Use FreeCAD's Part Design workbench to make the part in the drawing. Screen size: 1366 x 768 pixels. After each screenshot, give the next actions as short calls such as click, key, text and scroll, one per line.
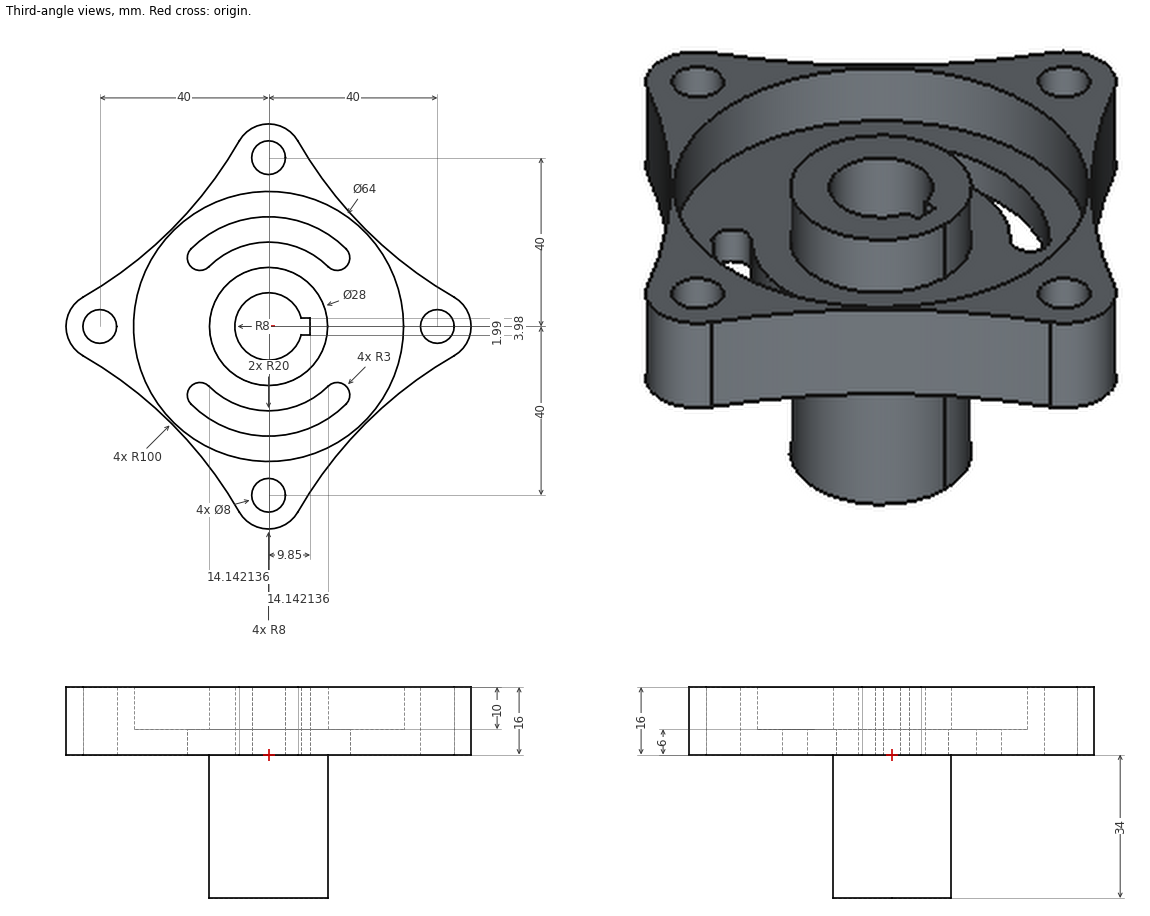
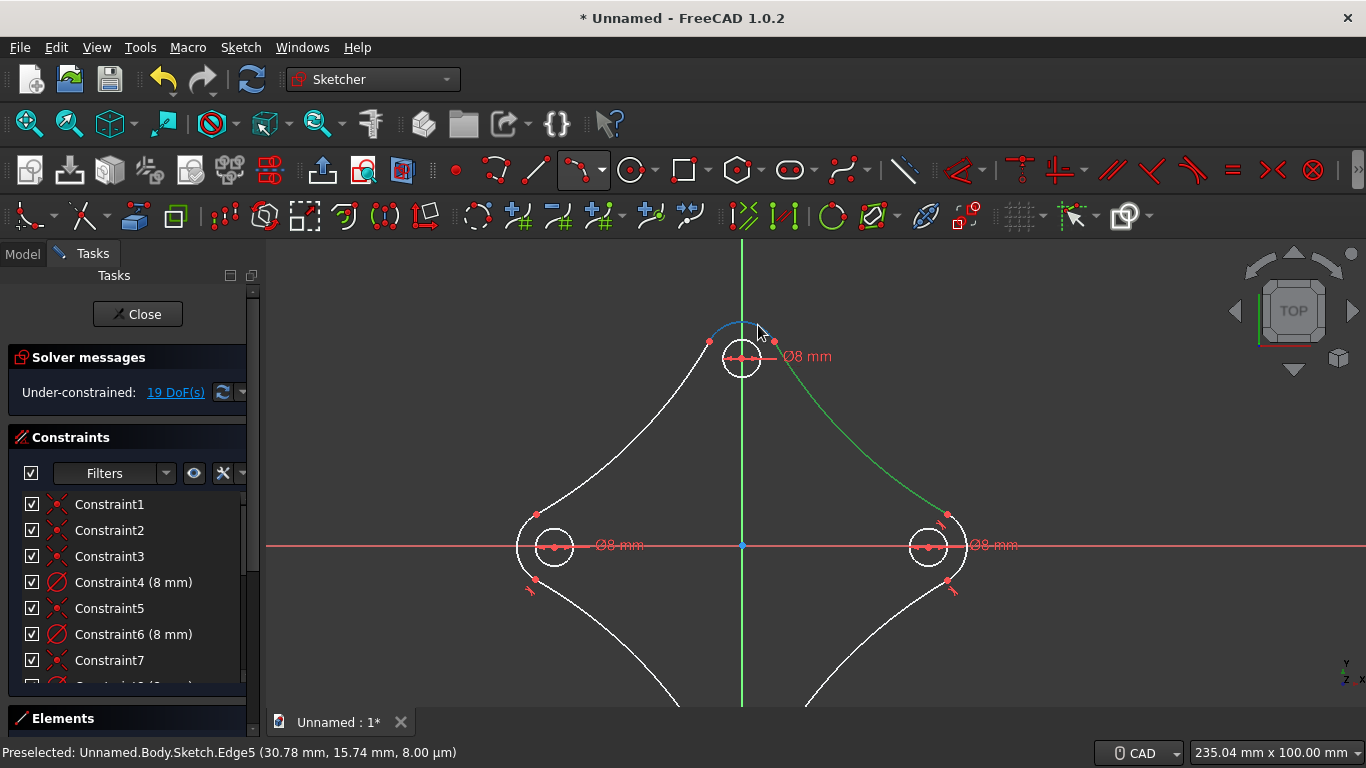
click(757, 325)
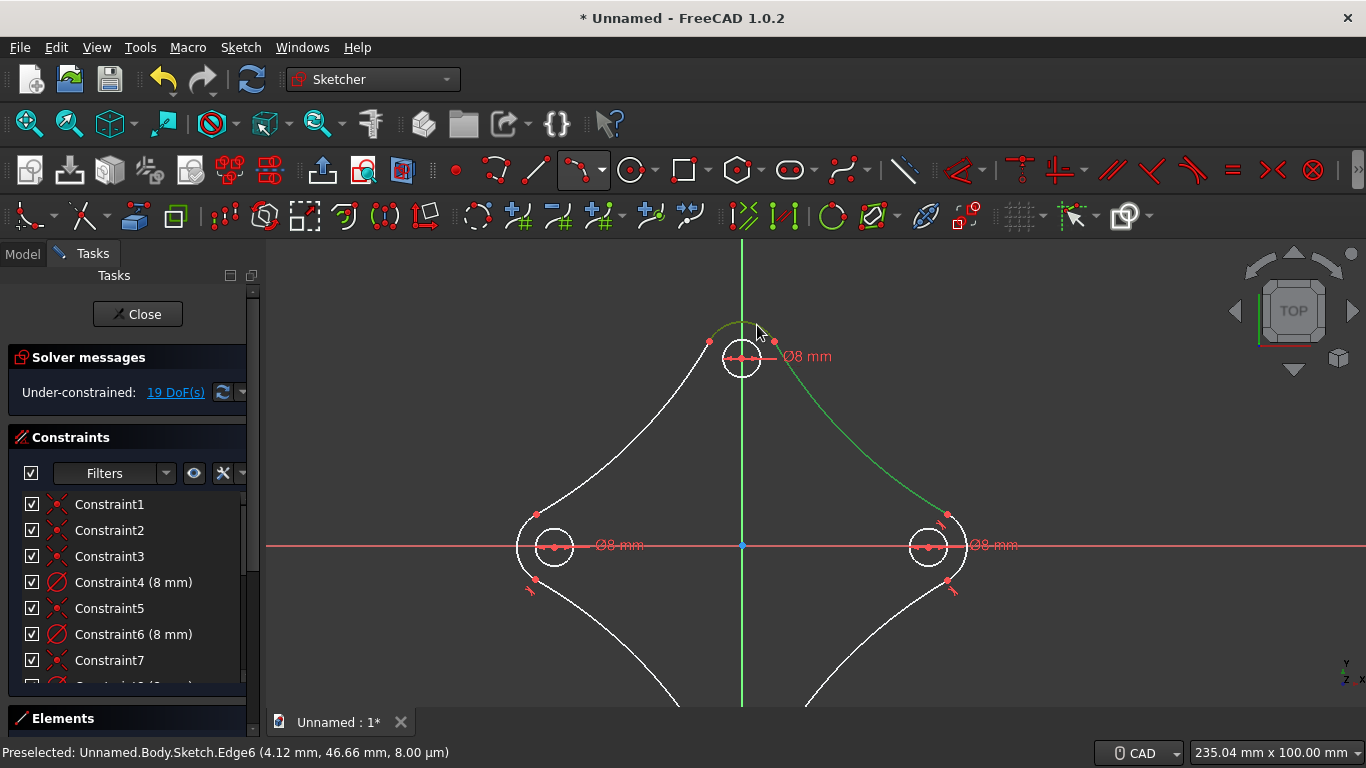
click(1194, 170)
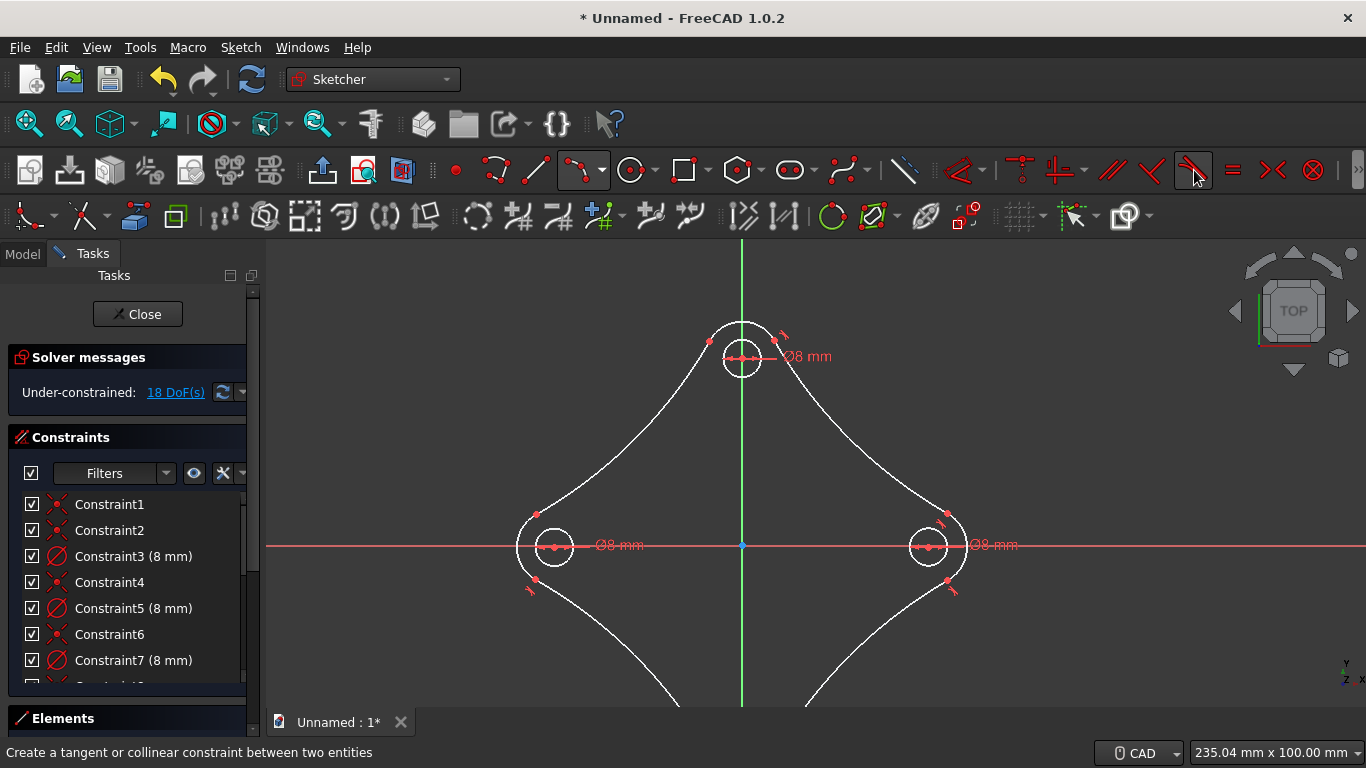
click(757, 325)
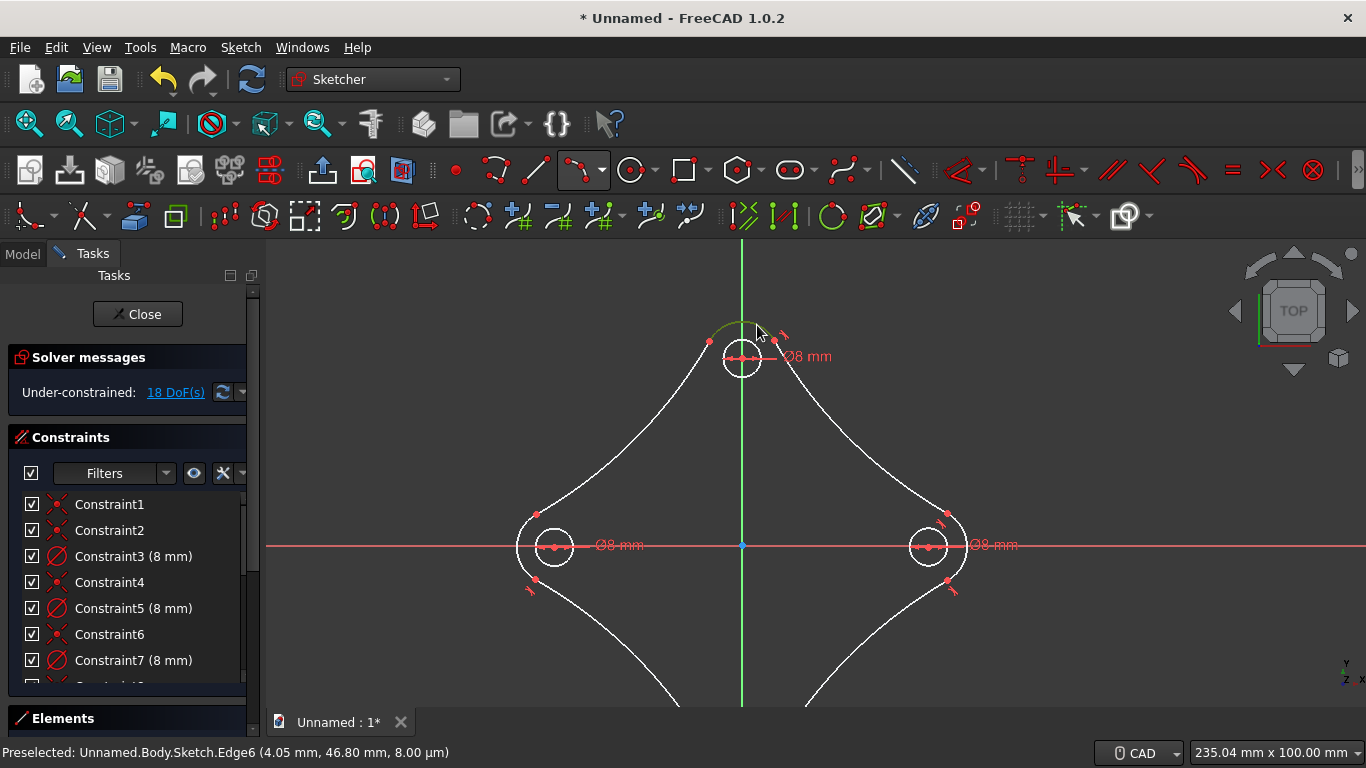
click(598, 473)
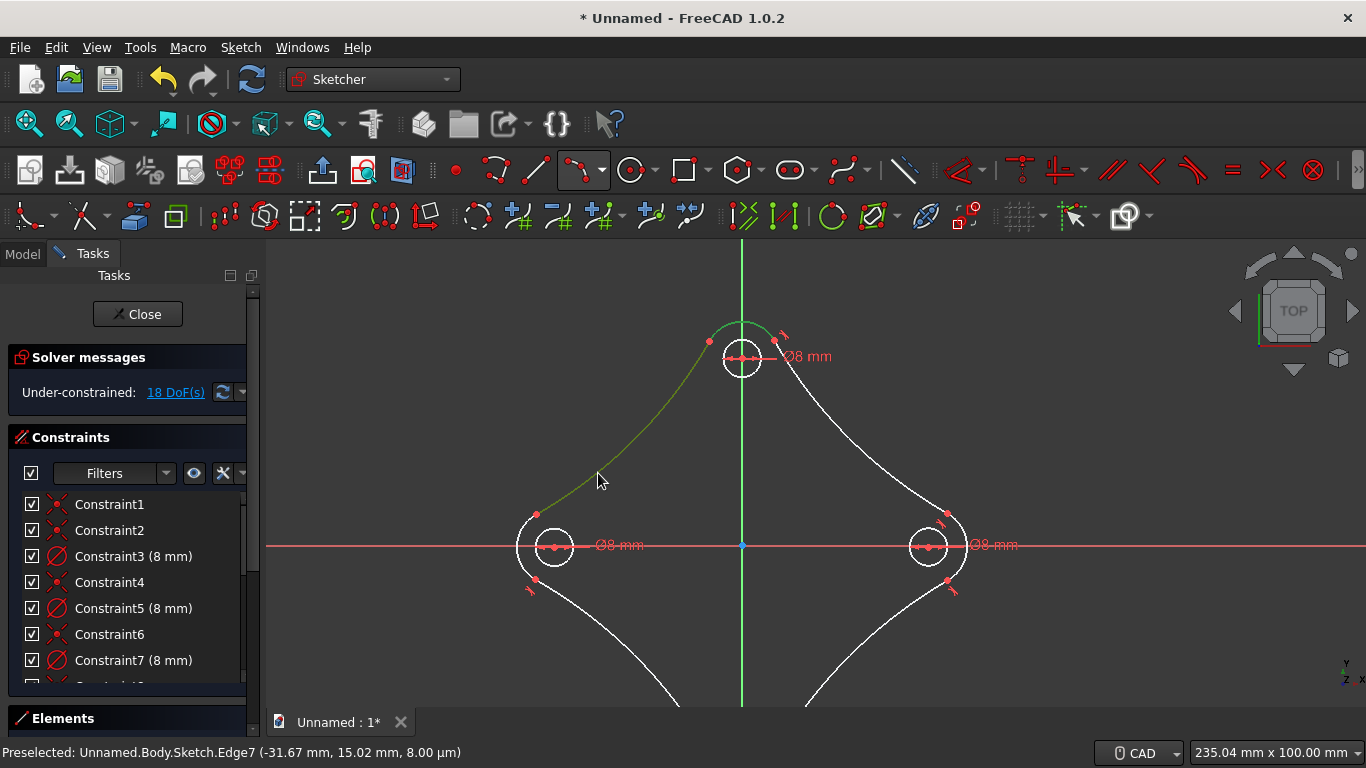
click(1194, 170)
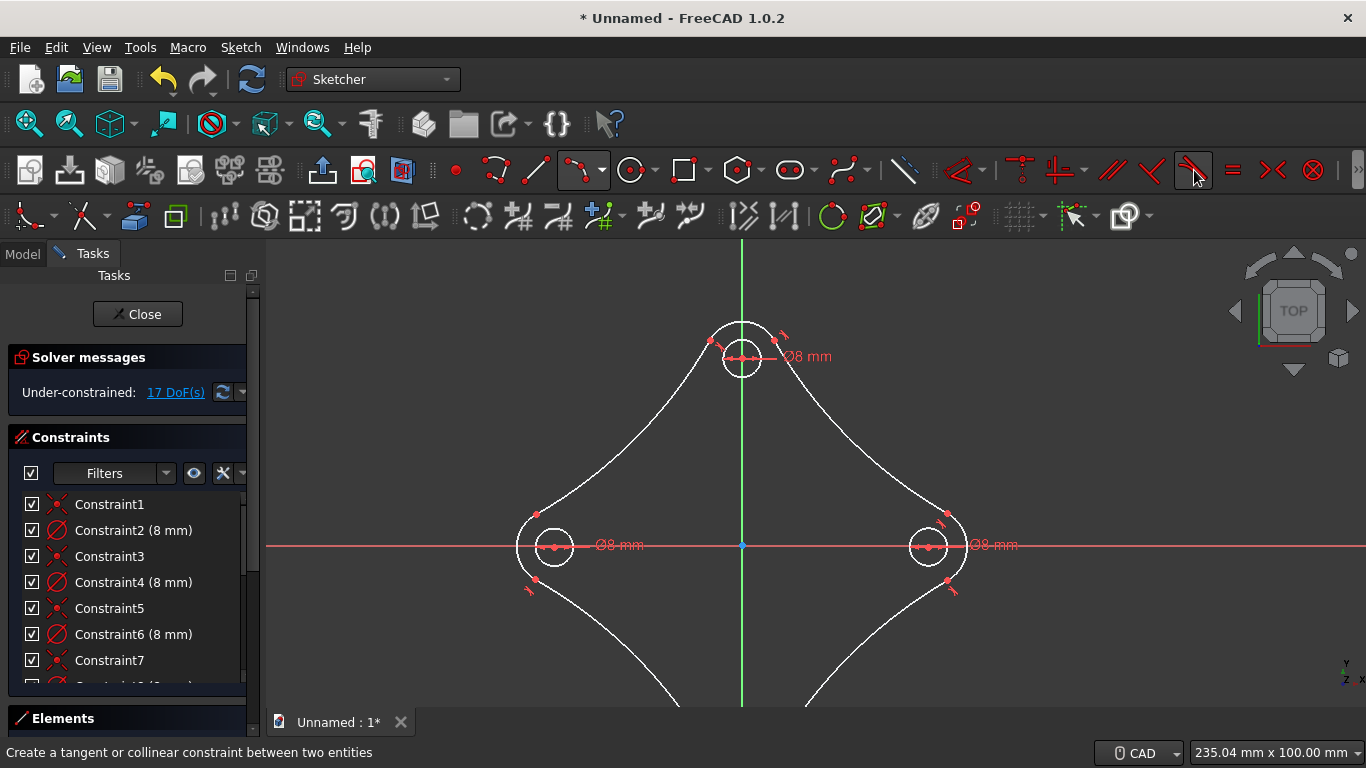
click(598, 472)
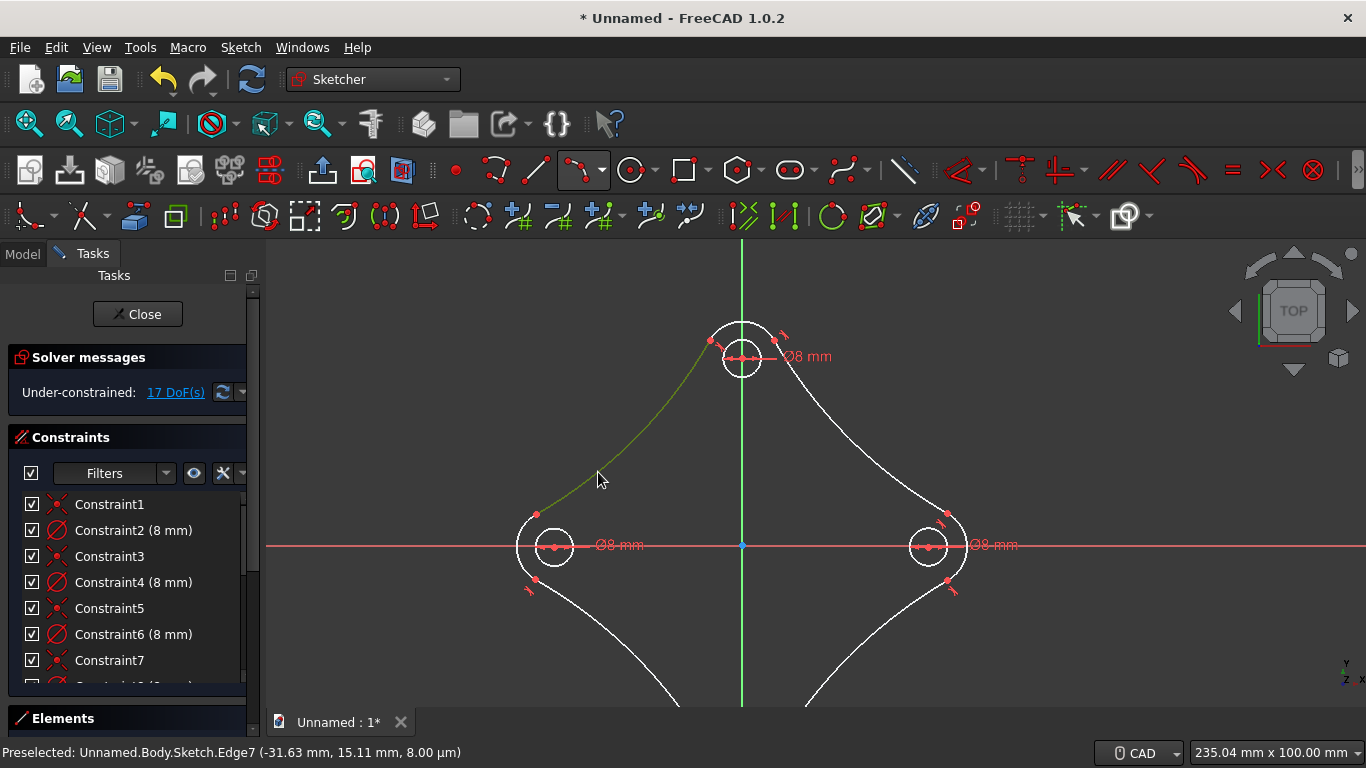
click(520, 531)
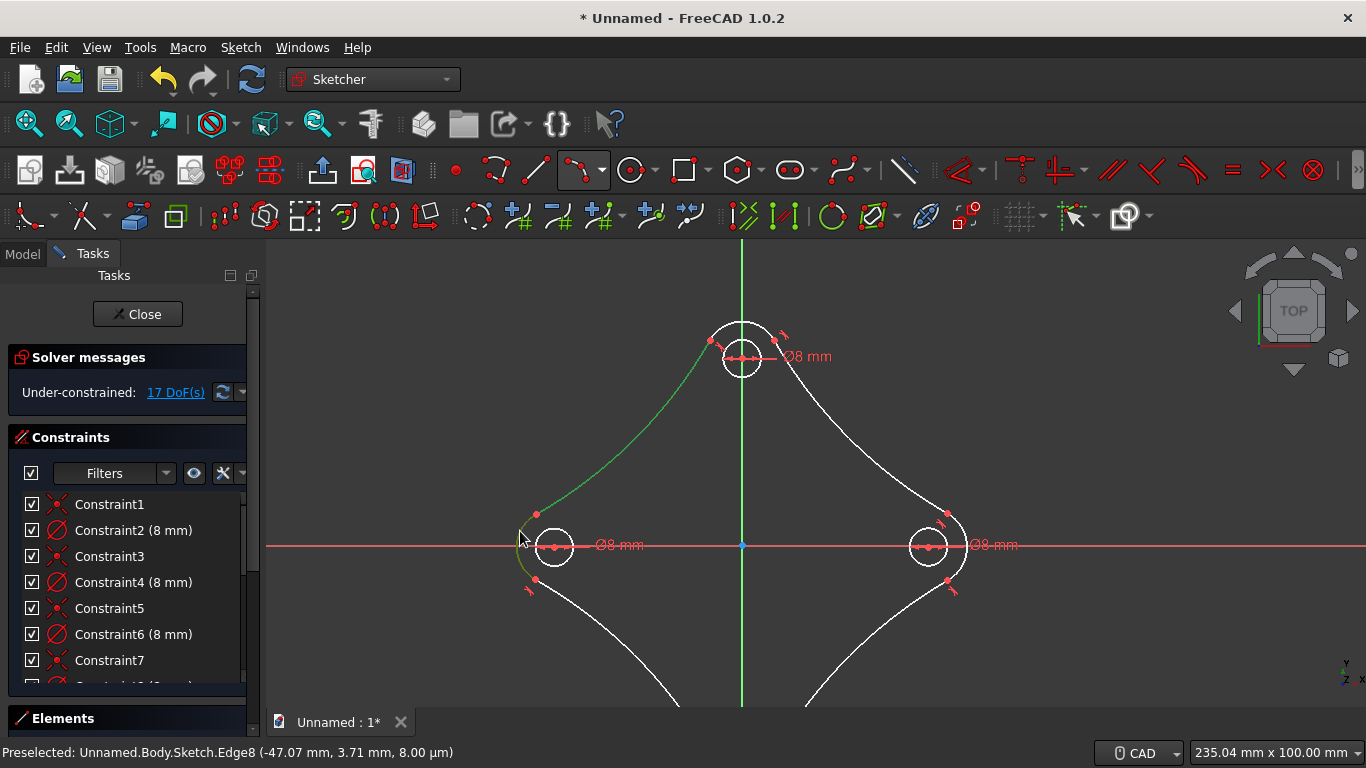
click(1194, 170)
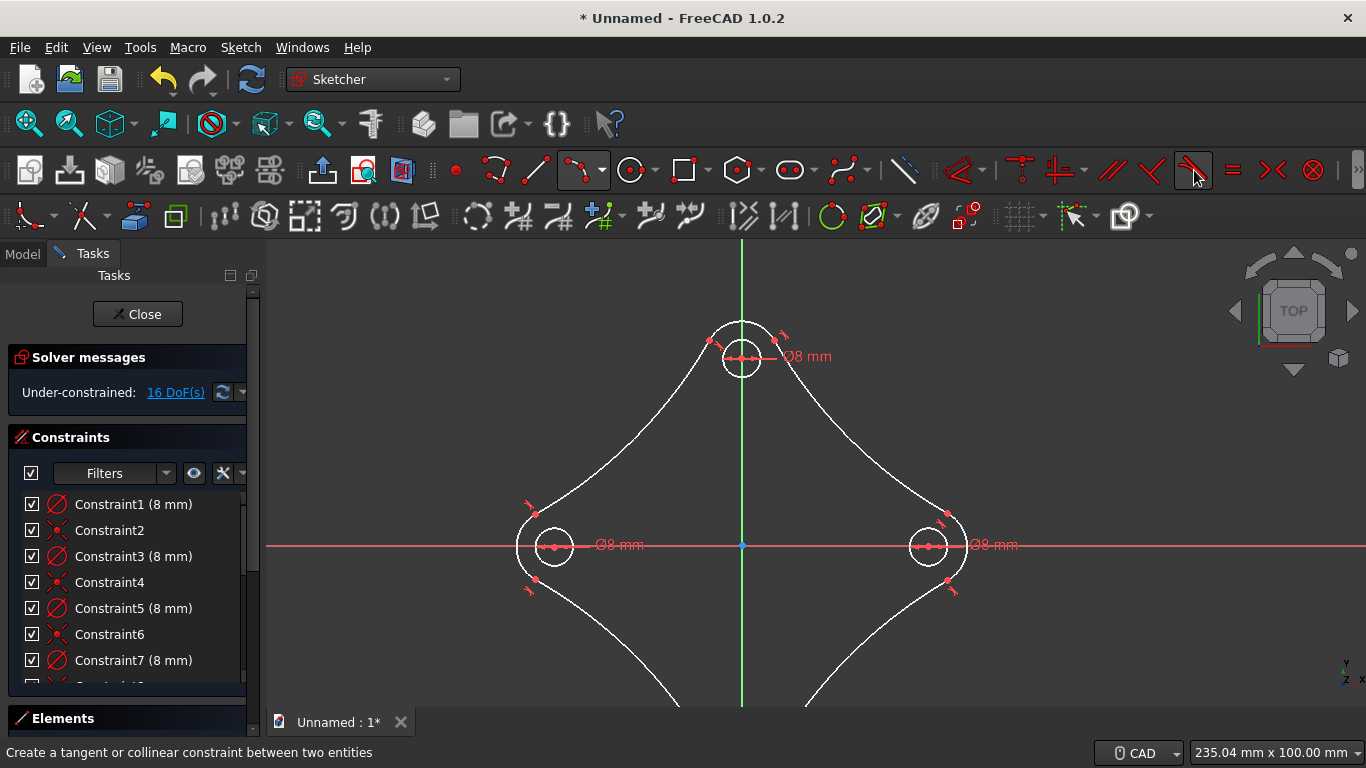
click(597, 622)